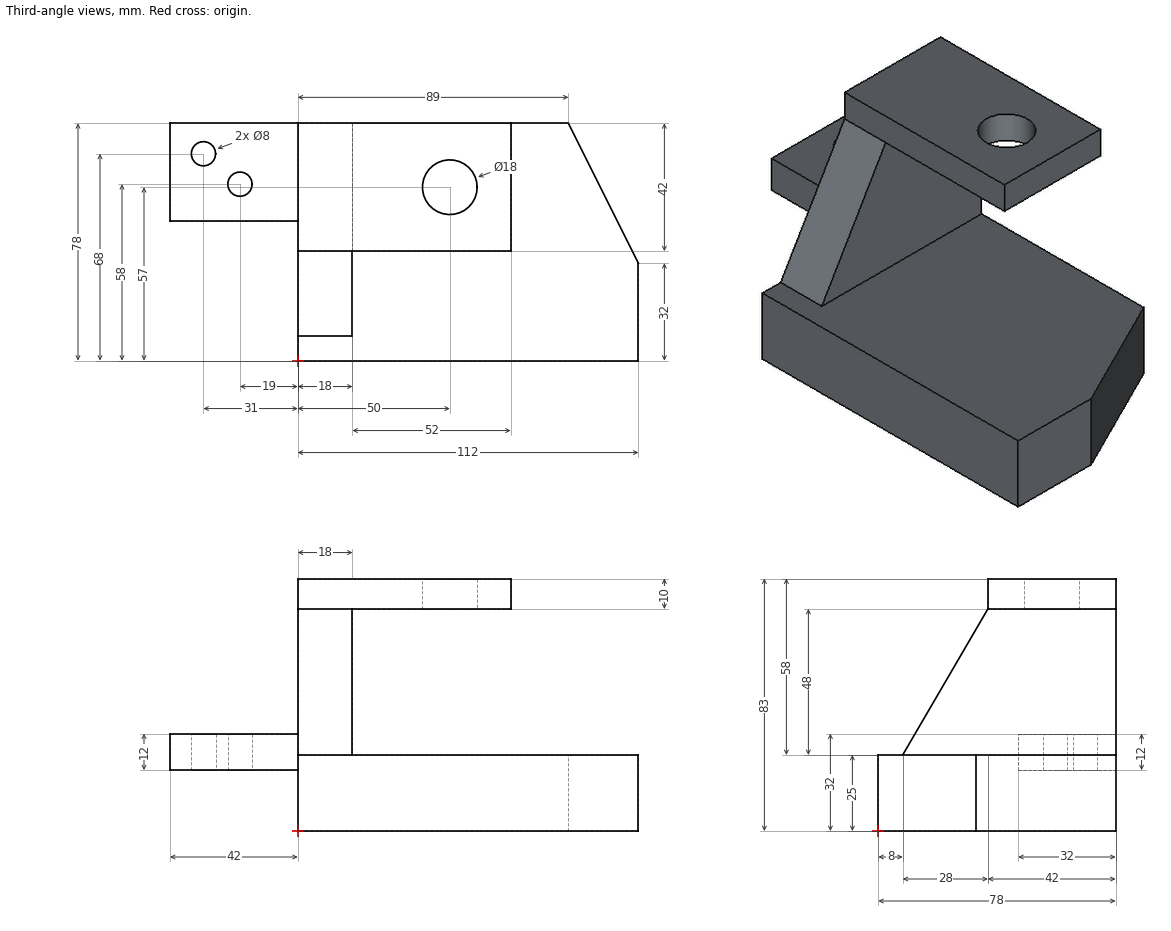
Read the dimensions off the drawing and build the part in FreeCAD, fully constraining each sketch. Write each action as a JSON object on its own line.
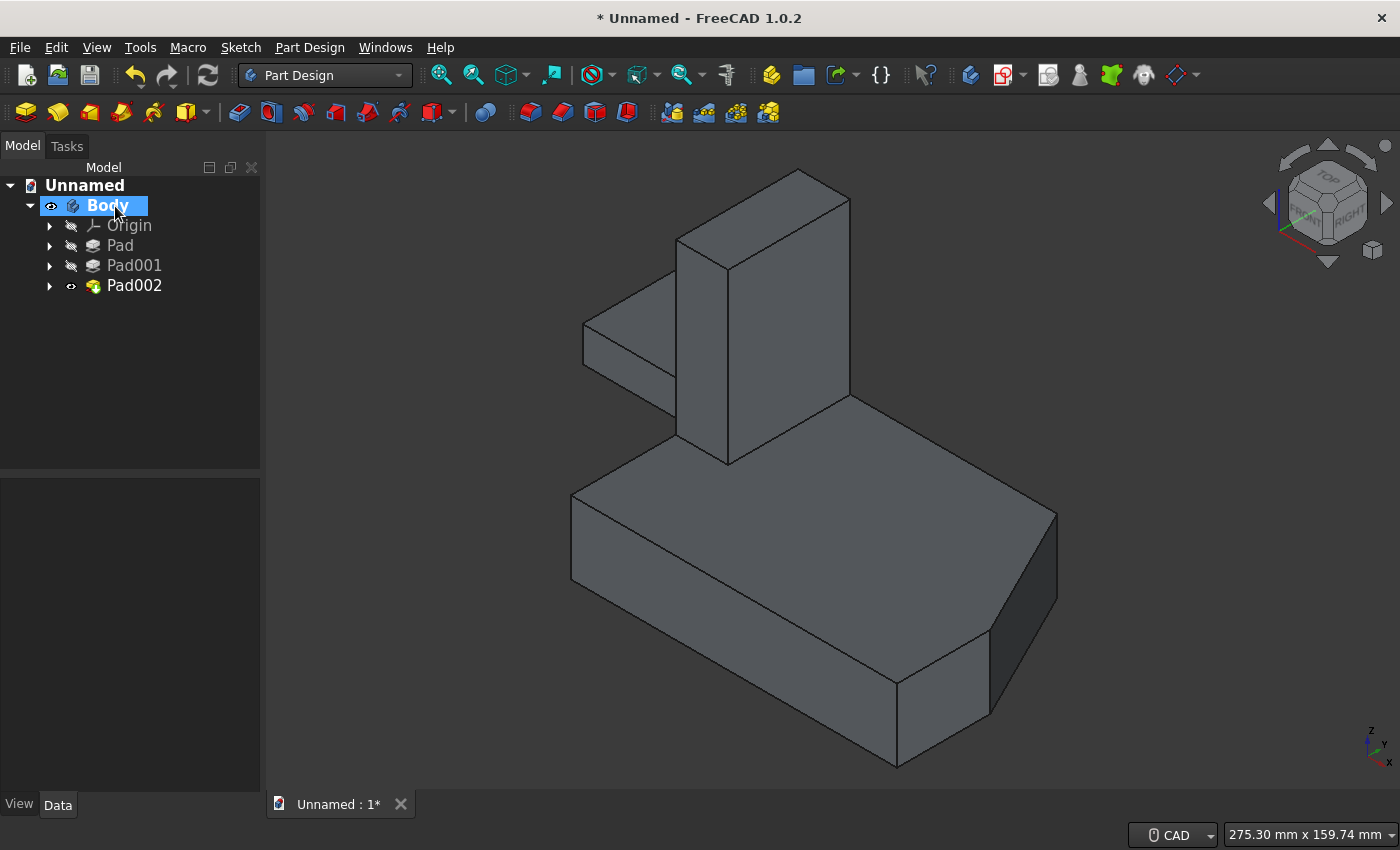
{"action": "key", "text": "v f"}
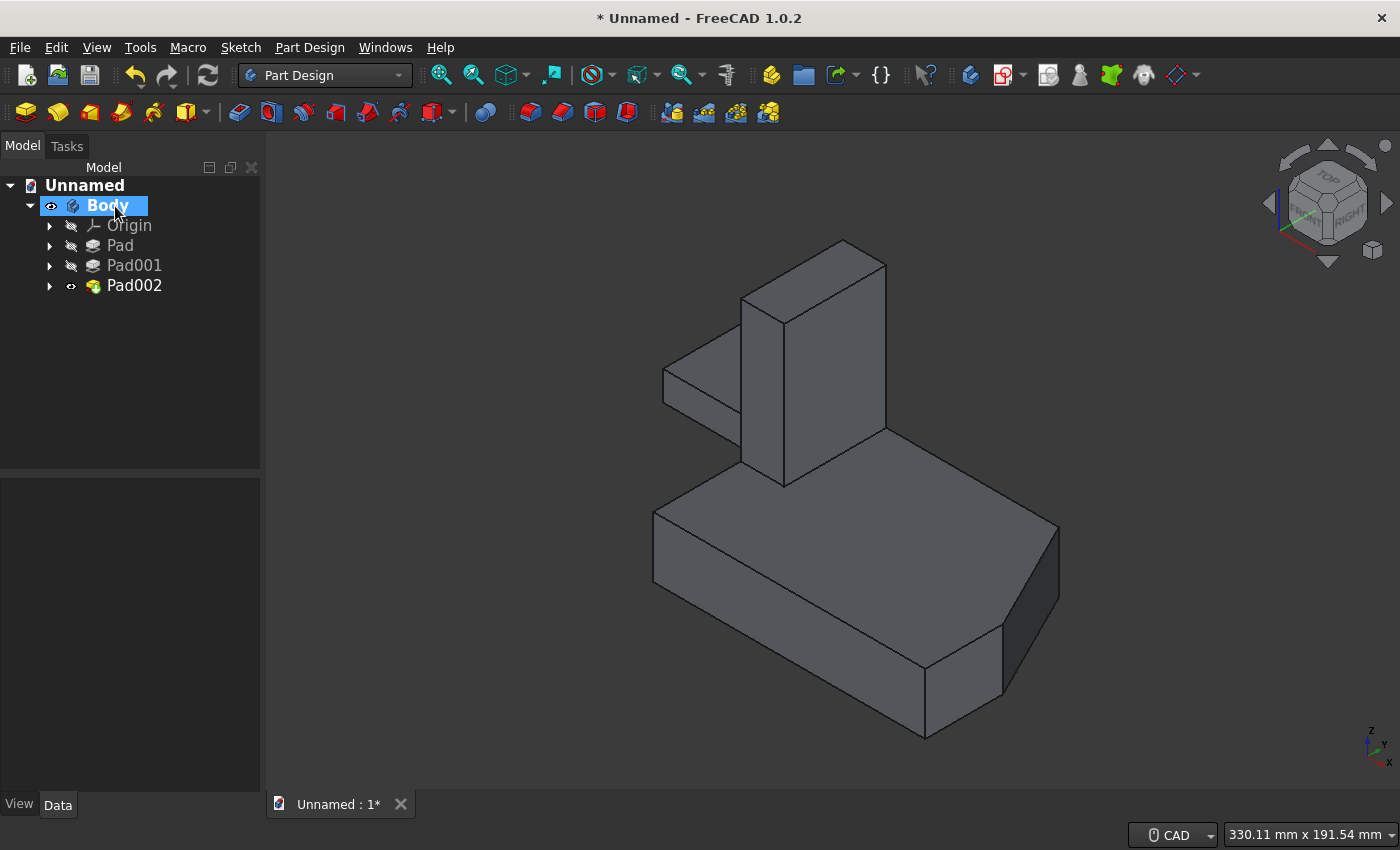
{"action": "left_click", "coordinate": [843, 264]}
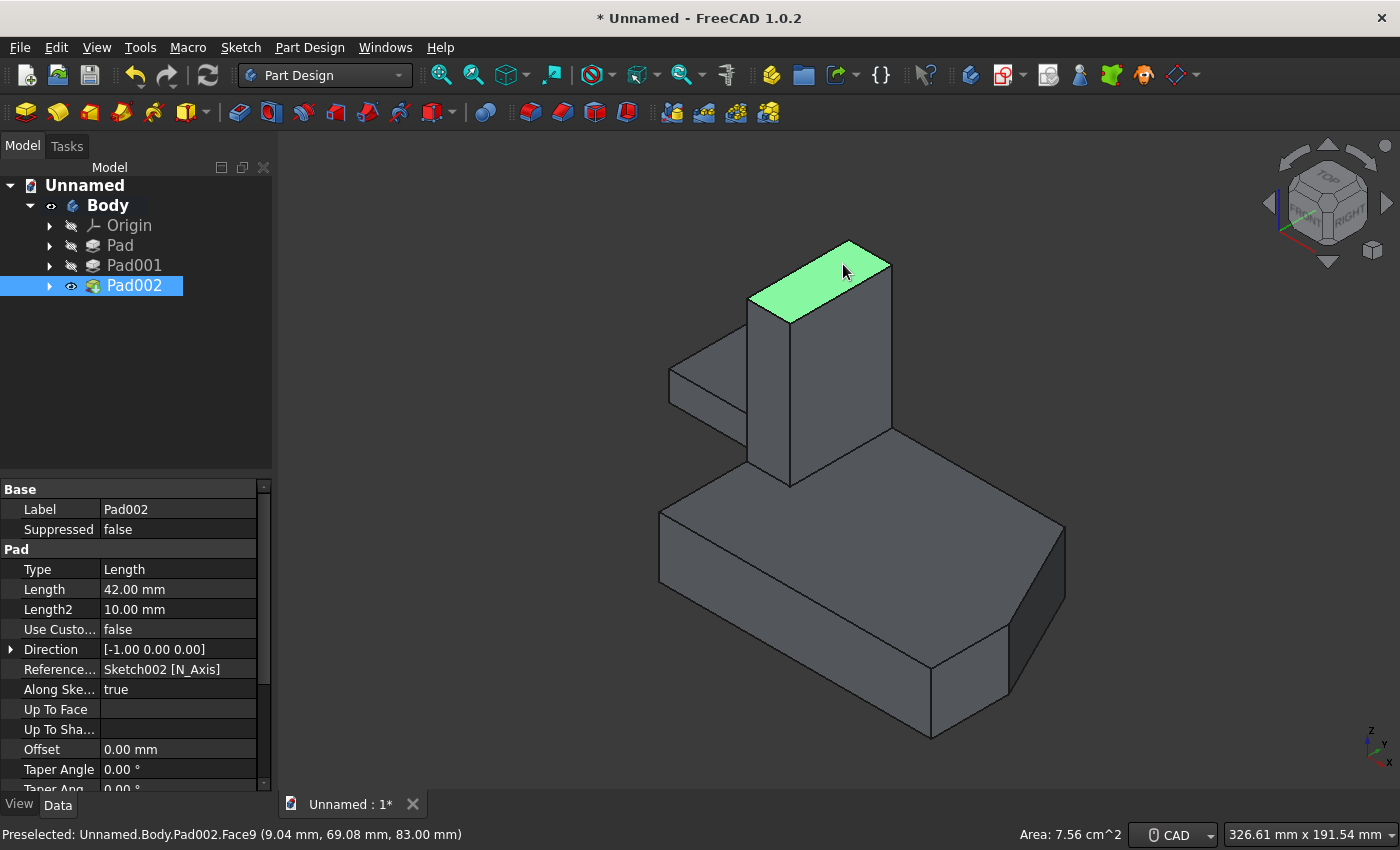
{"action": "left_click", "coordinate": [1004, 76]}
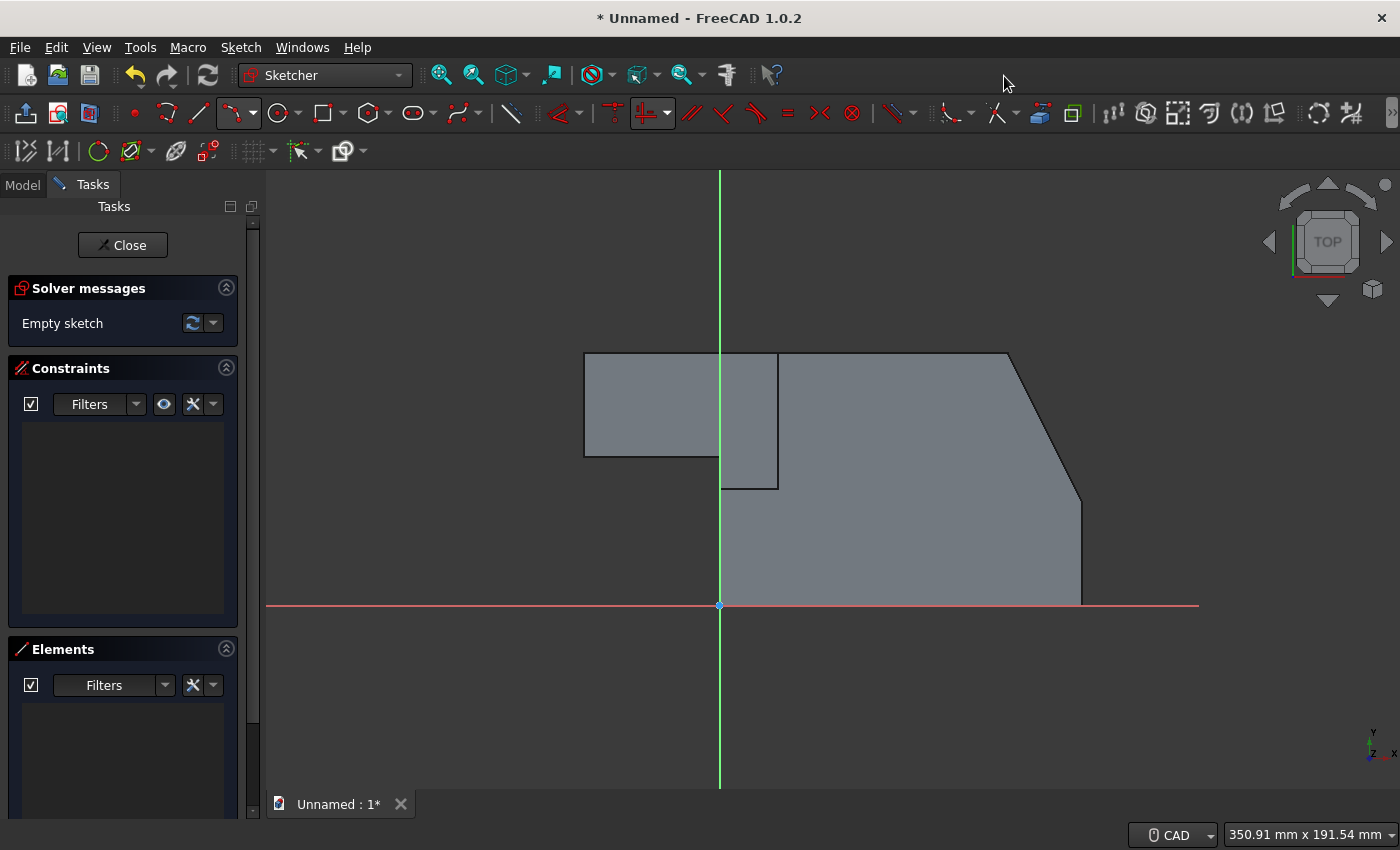
{"action": "scroll", "coordinate": [972, 479], "scroll_direction": "up", "scroll_amount": 2}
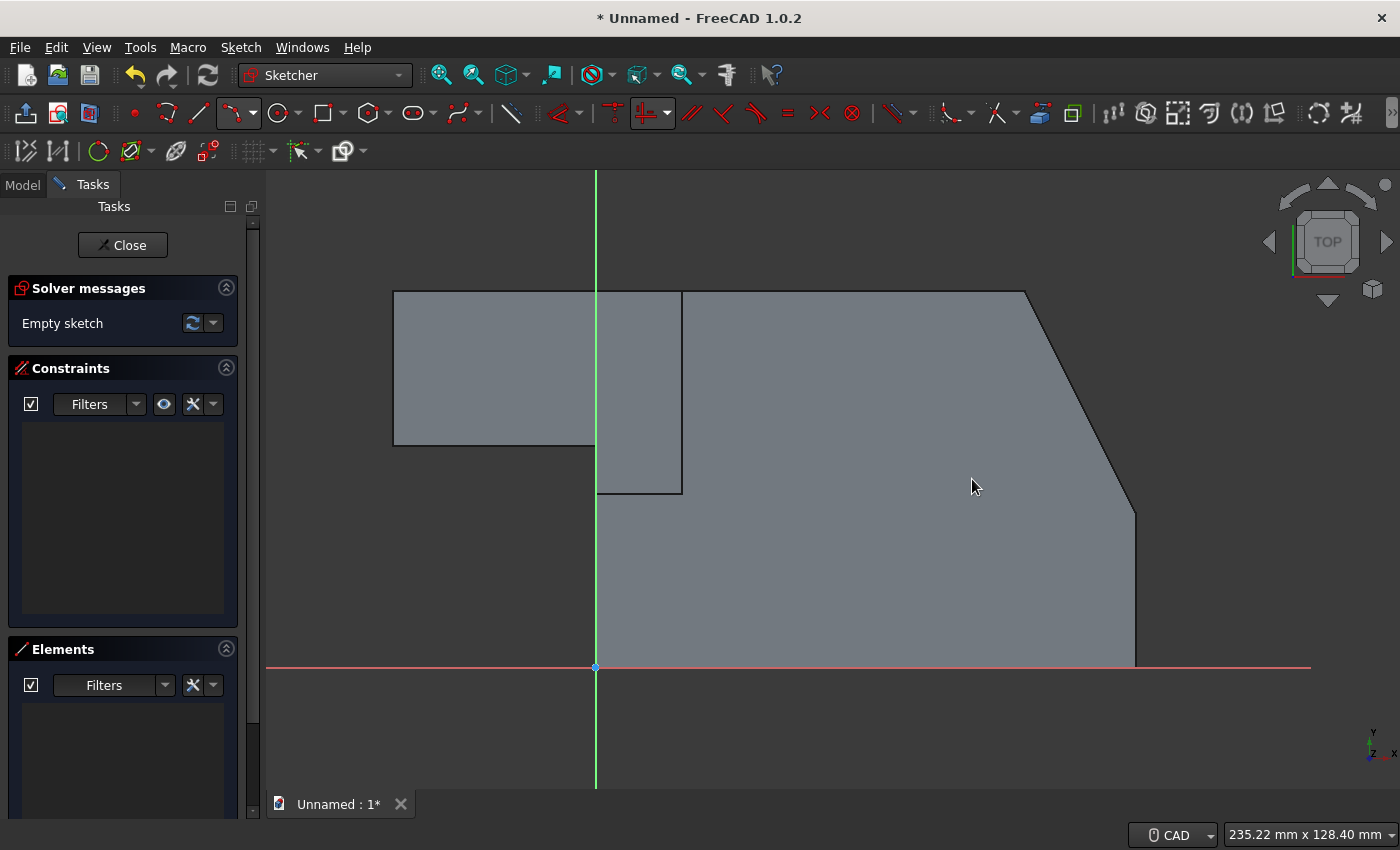
{"action": "key", "text": "g r"}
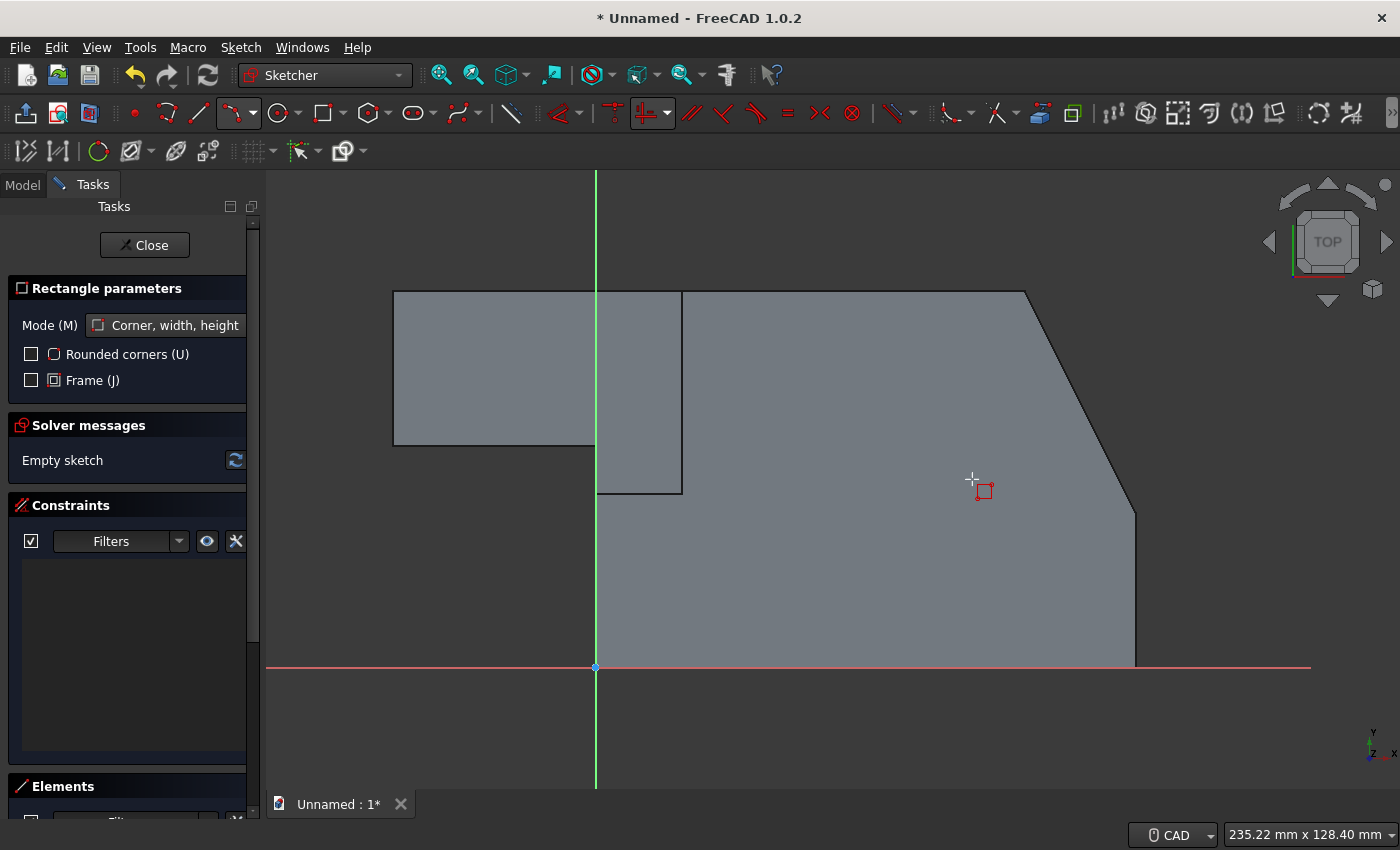
{"action": "left_click", "coordinate": [682, 291]}
{"action": "mouse_move", "coordinate": [933, 494]}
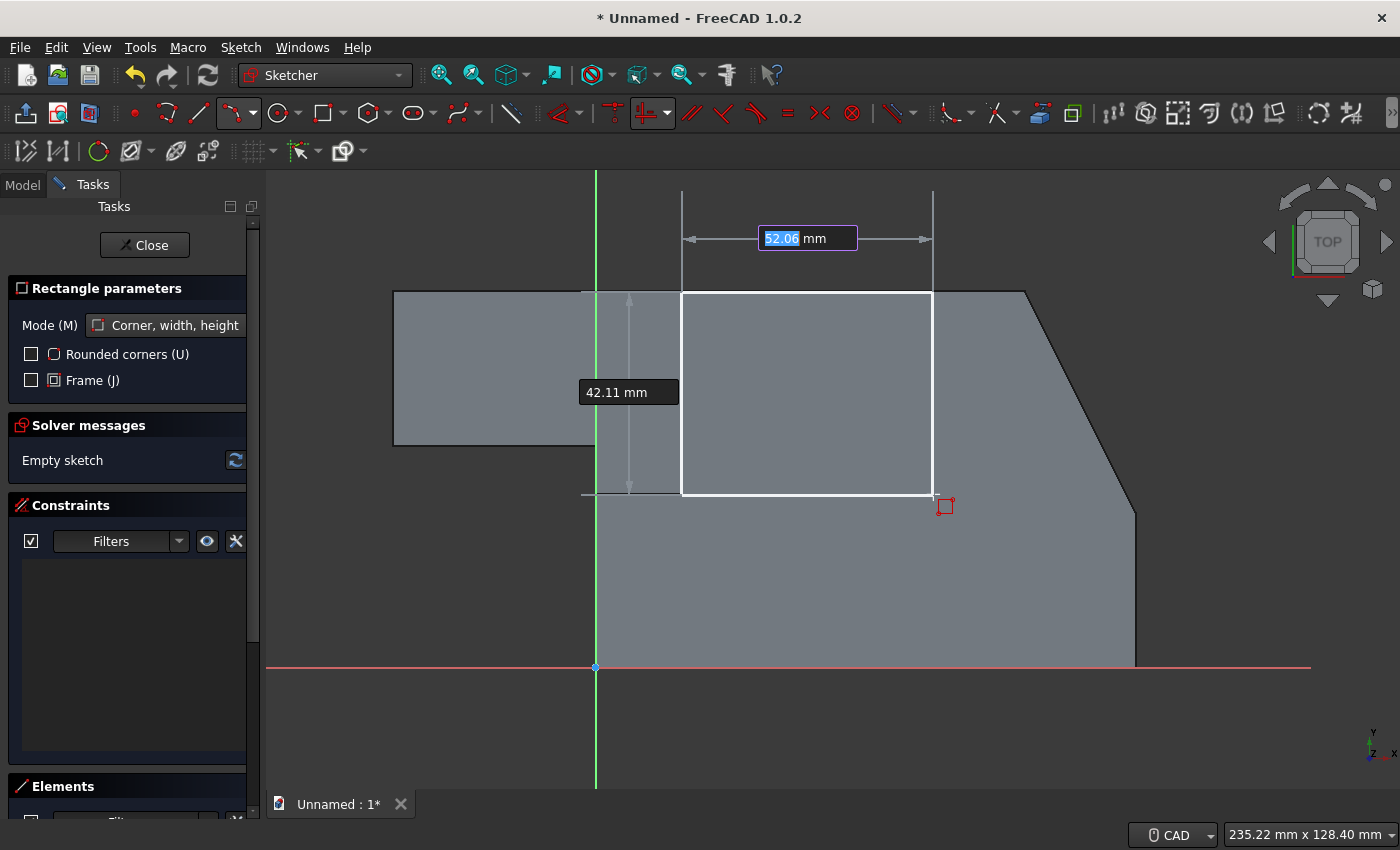
{"action": "type", "text": "52"}
{"action": "key", "text": "Tab"}
{"action": "type", "text": "42"}
{"action": "key", "text": "Return"}
{"action": "key", "text": "Escape"}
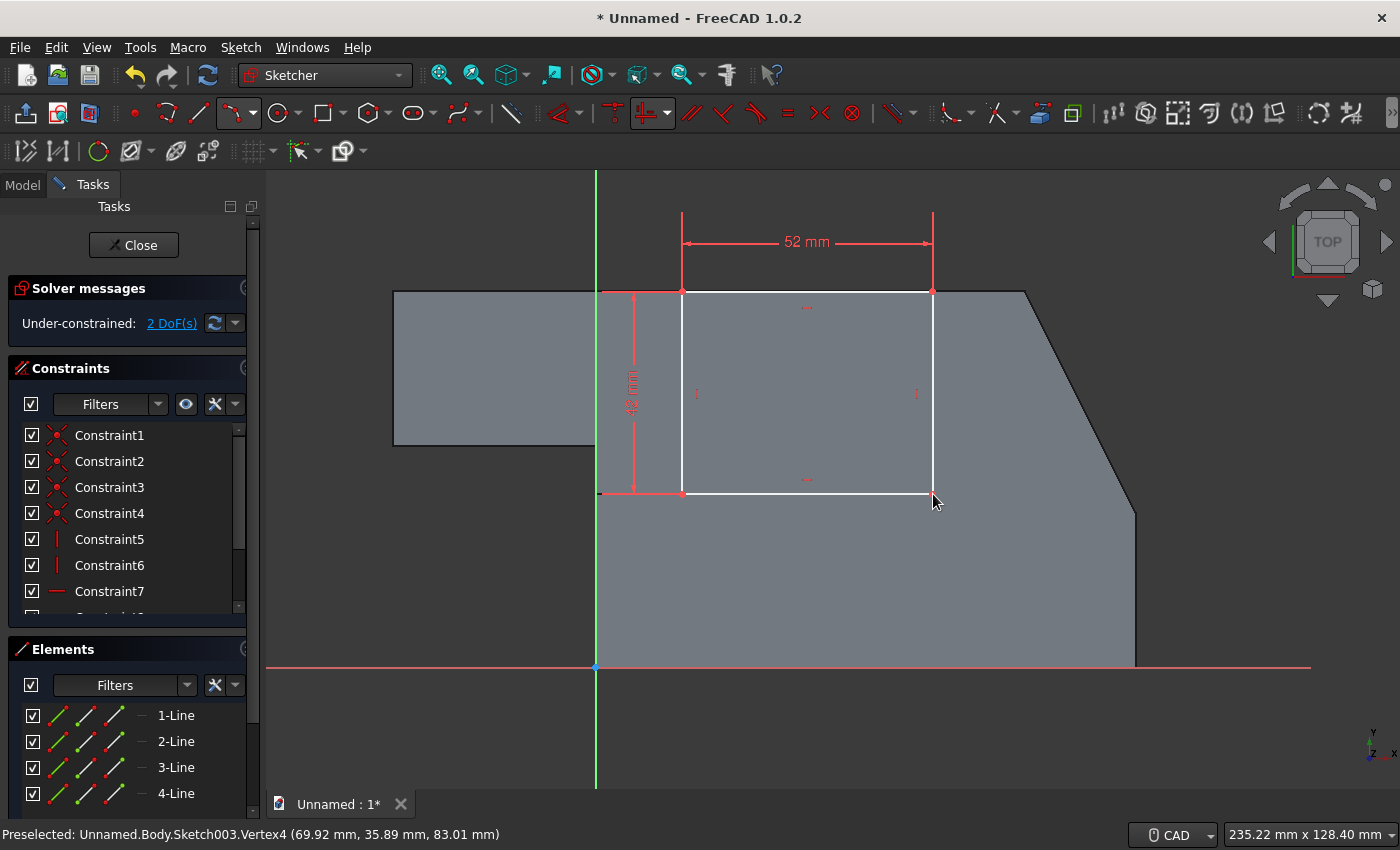
{"action": "key", "text": "d"}